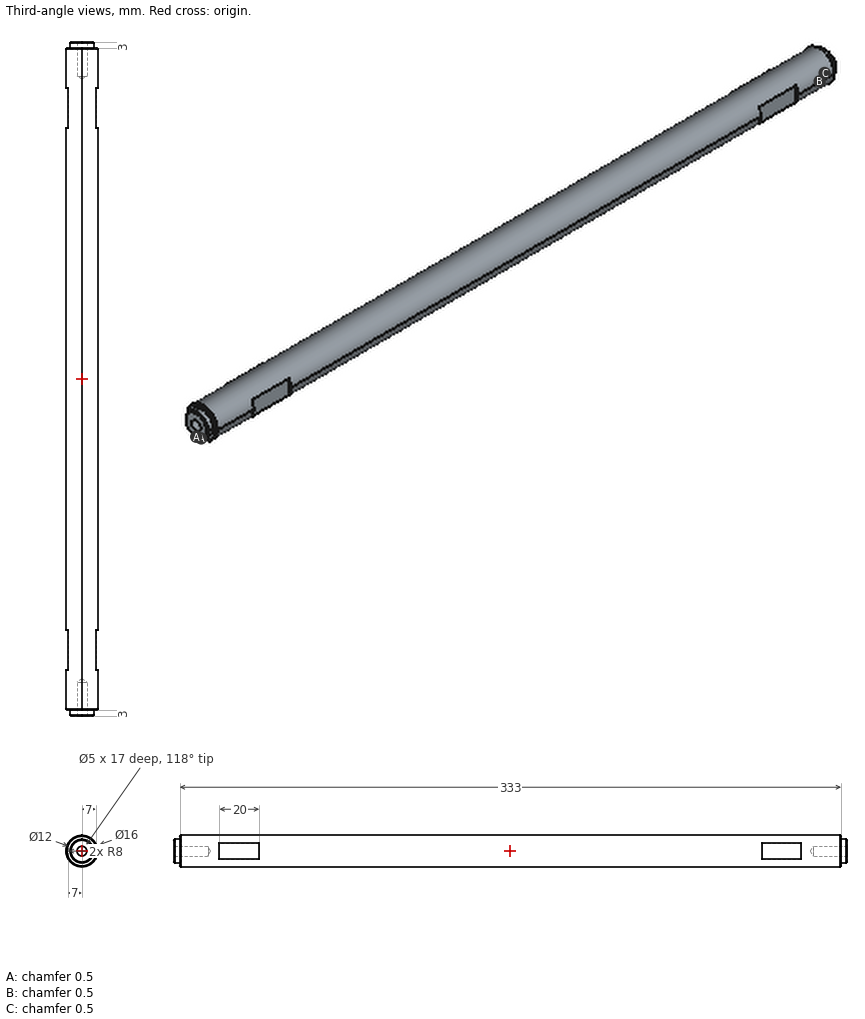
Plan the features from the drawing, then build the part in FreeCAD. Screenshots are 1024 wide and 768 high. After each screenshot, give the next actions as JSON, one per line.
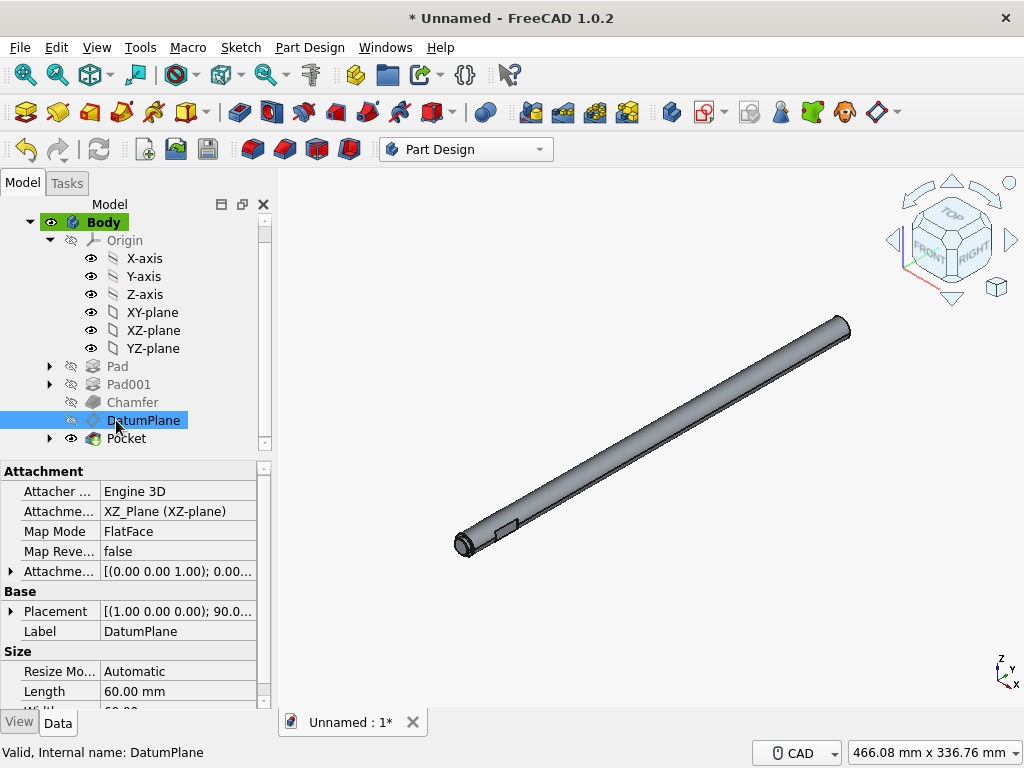
{"action": "key", "text": "2"}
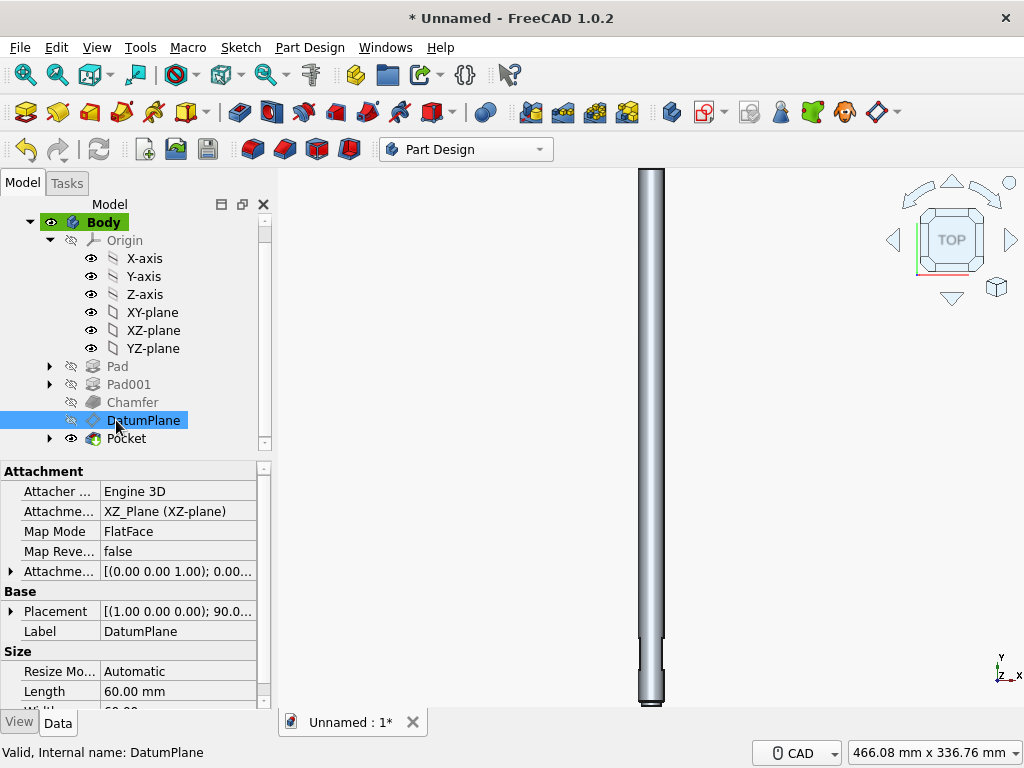
{"action": "left_click", "coordinate": [136, 330]}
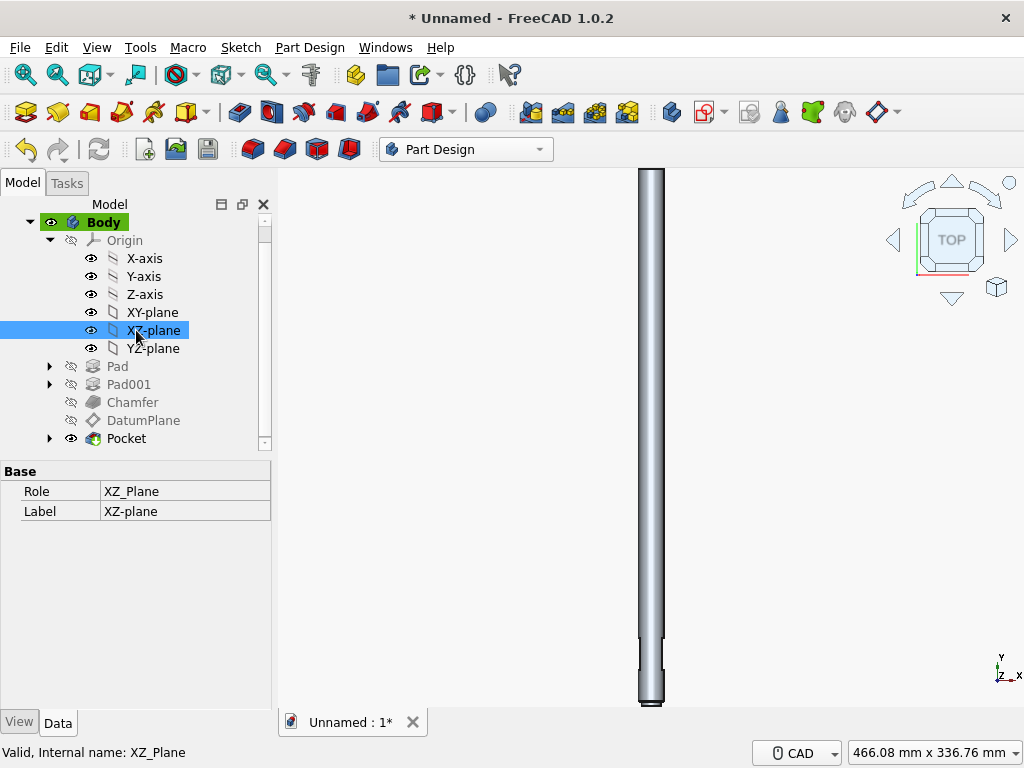
{"action": "left_click", "coordinate": [878, 112]}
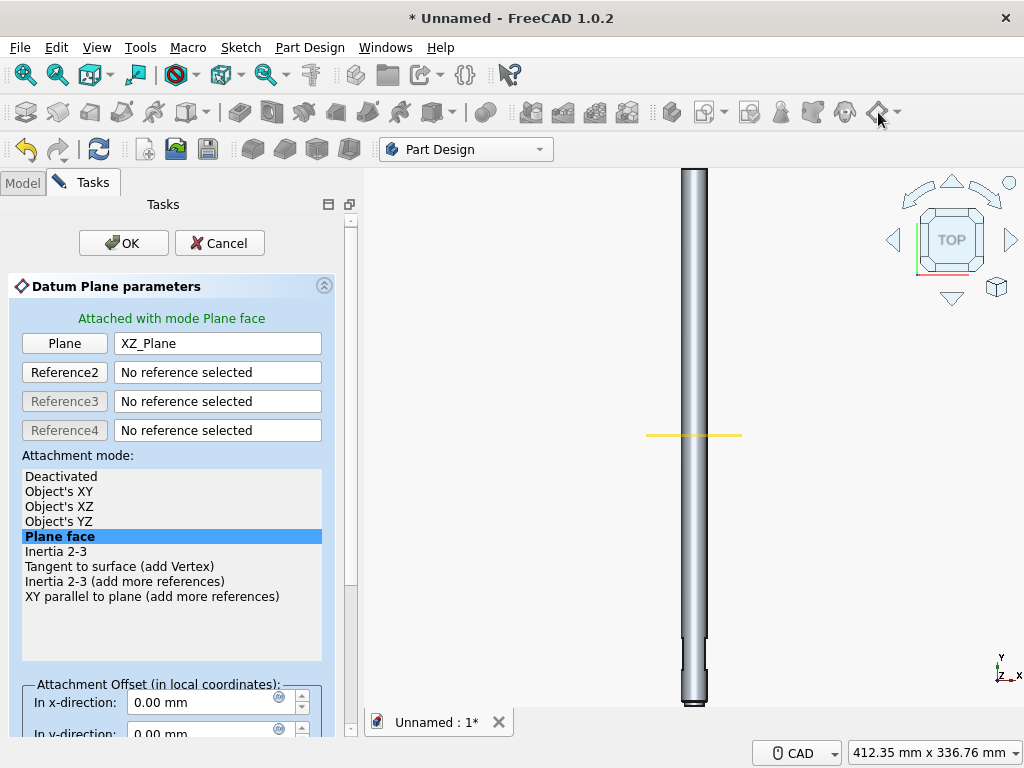
{"action": "scroll", "coordinate": [351, 475], "scroll_direction": "down", "scroll_amount": 2}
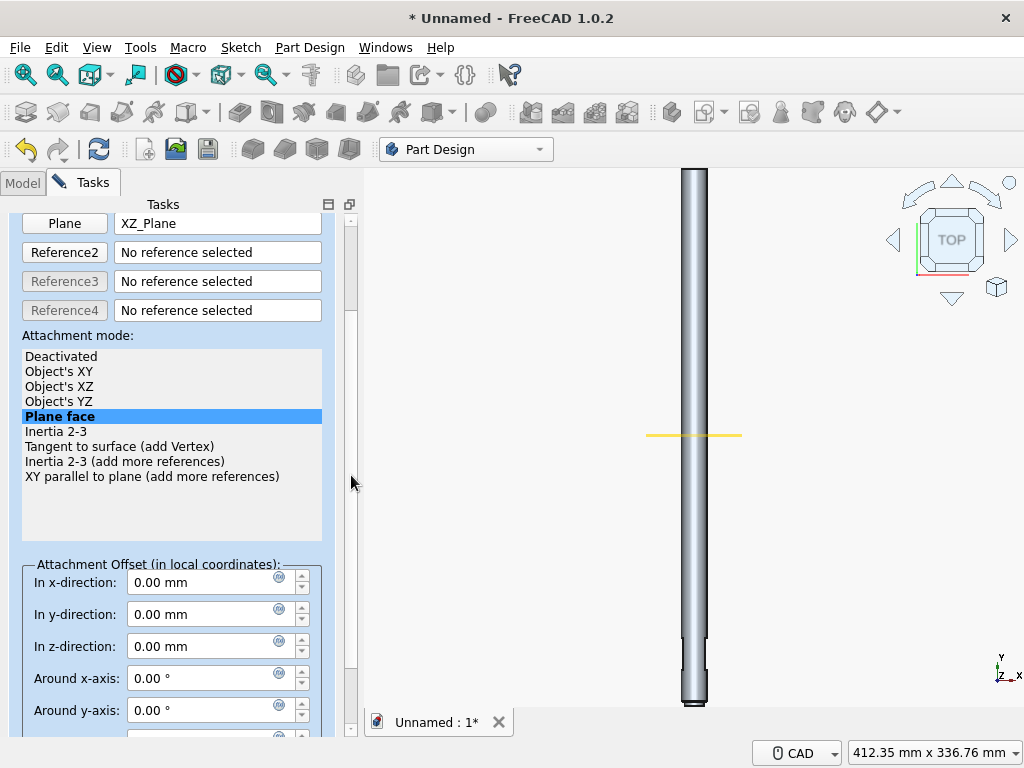
{"action": "triple_click", "coordinate": [210, 646]}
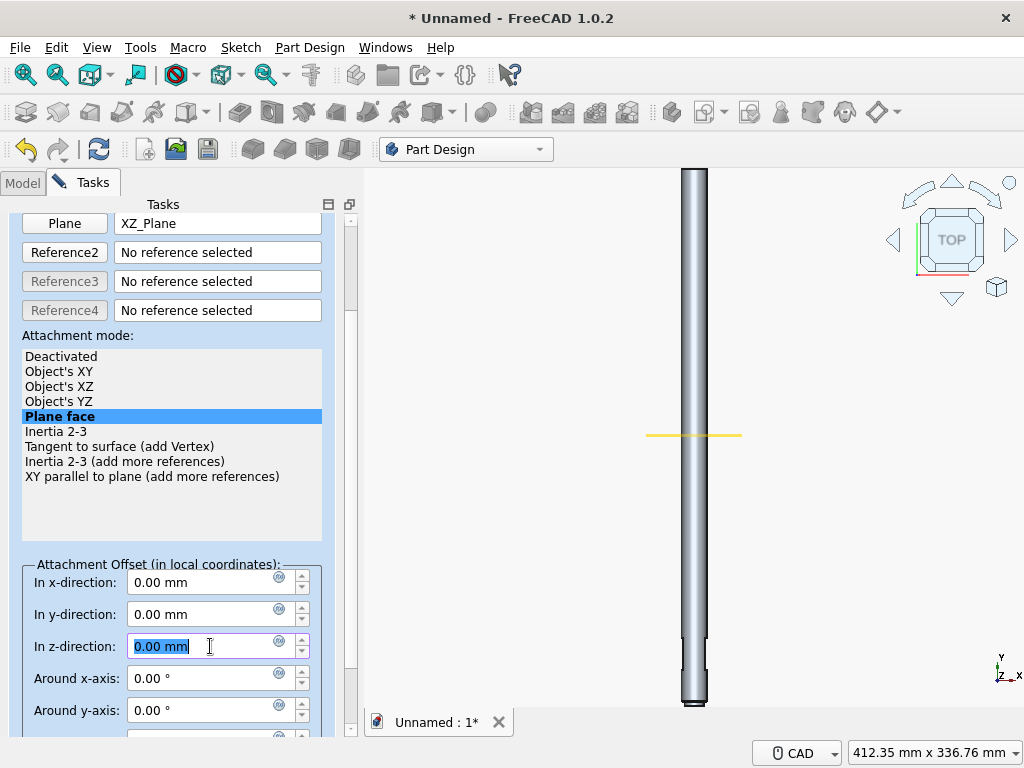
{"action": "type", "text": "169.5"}
{"action": "key", "text": "Tab"}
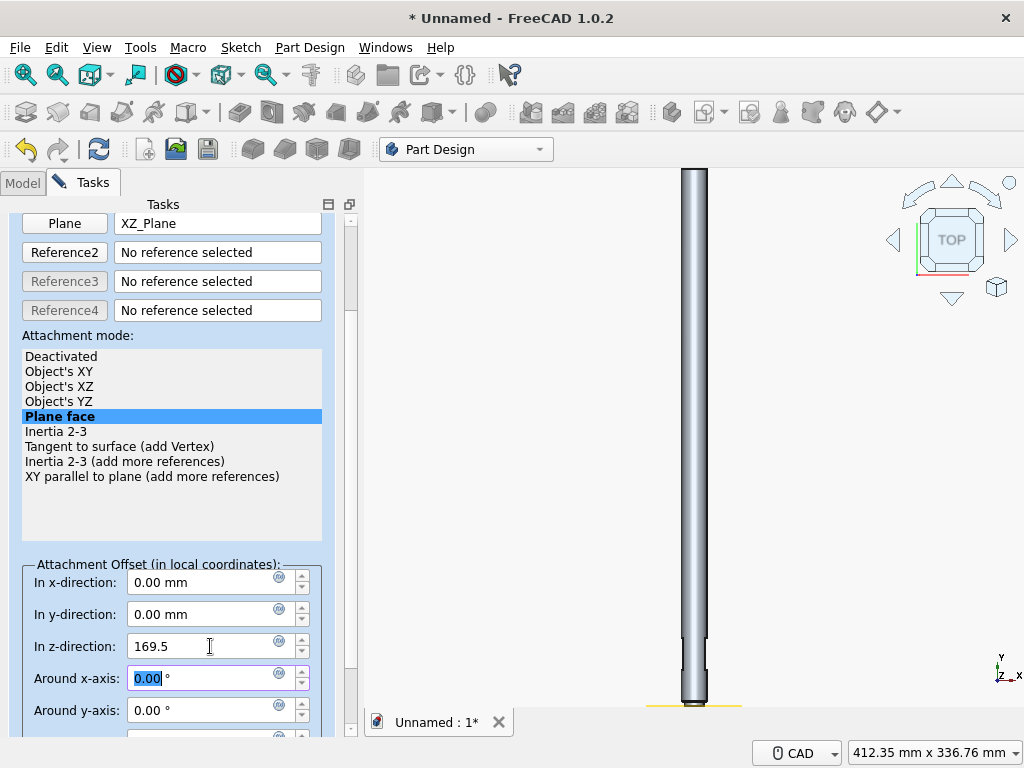
{"action": "scroll", "coordinate": [351, 475], "scroll_direction": "up", "scroll_amount": 3}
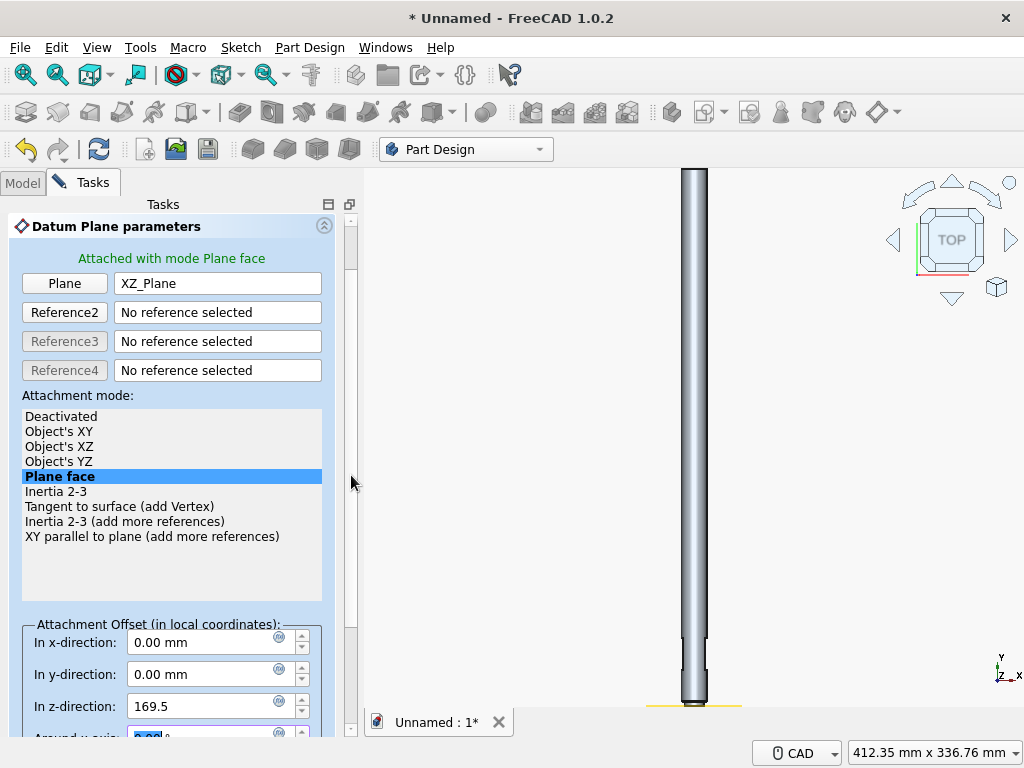
{"action": "left_click", "coordinate": [124, 243]}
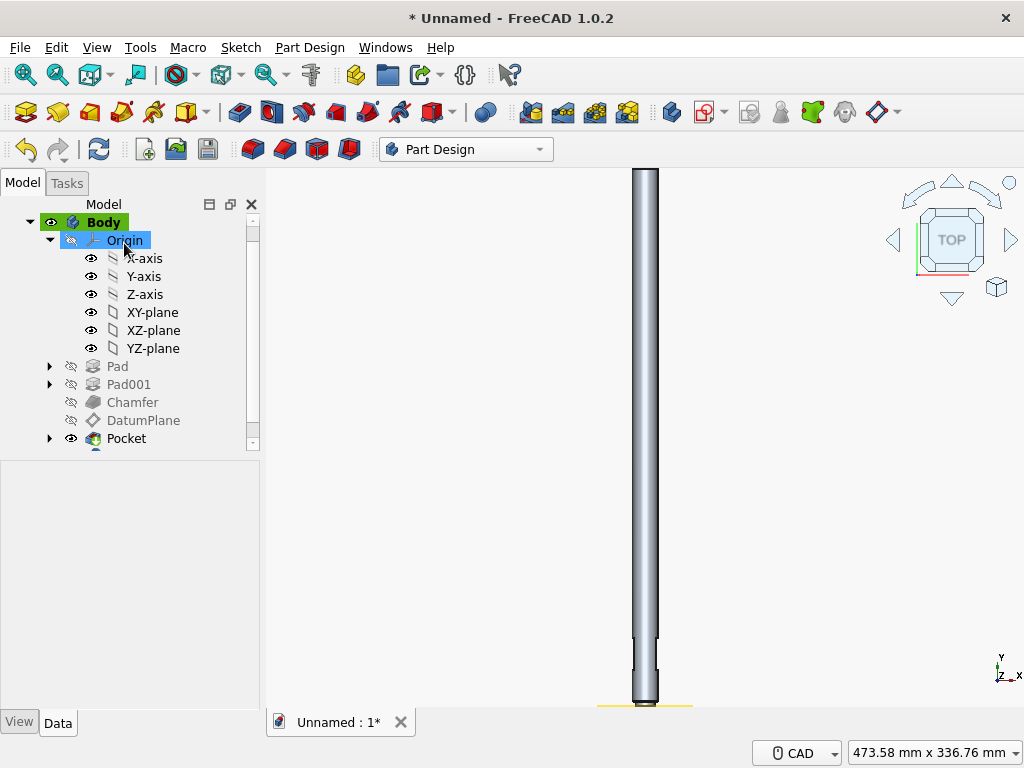
{"action": "scroll", "coordinate": [120, 326], "scroll_direction": "down", "scroll_amount": 3}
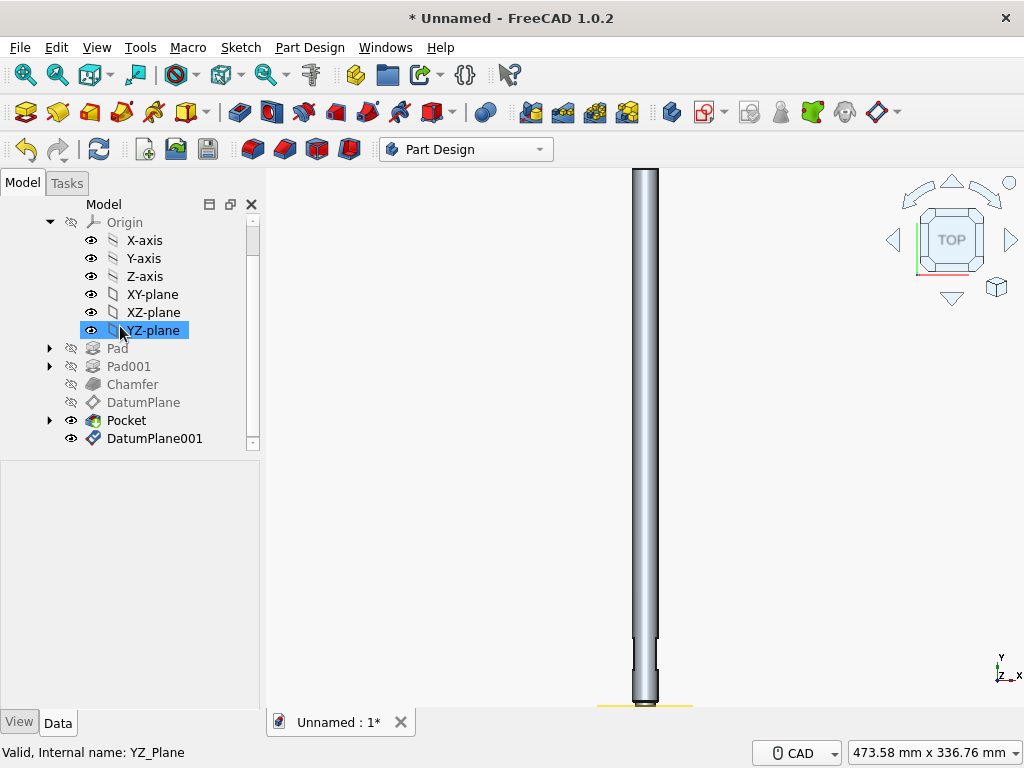
{"action": "left_click", "coordinate": [116, 438]}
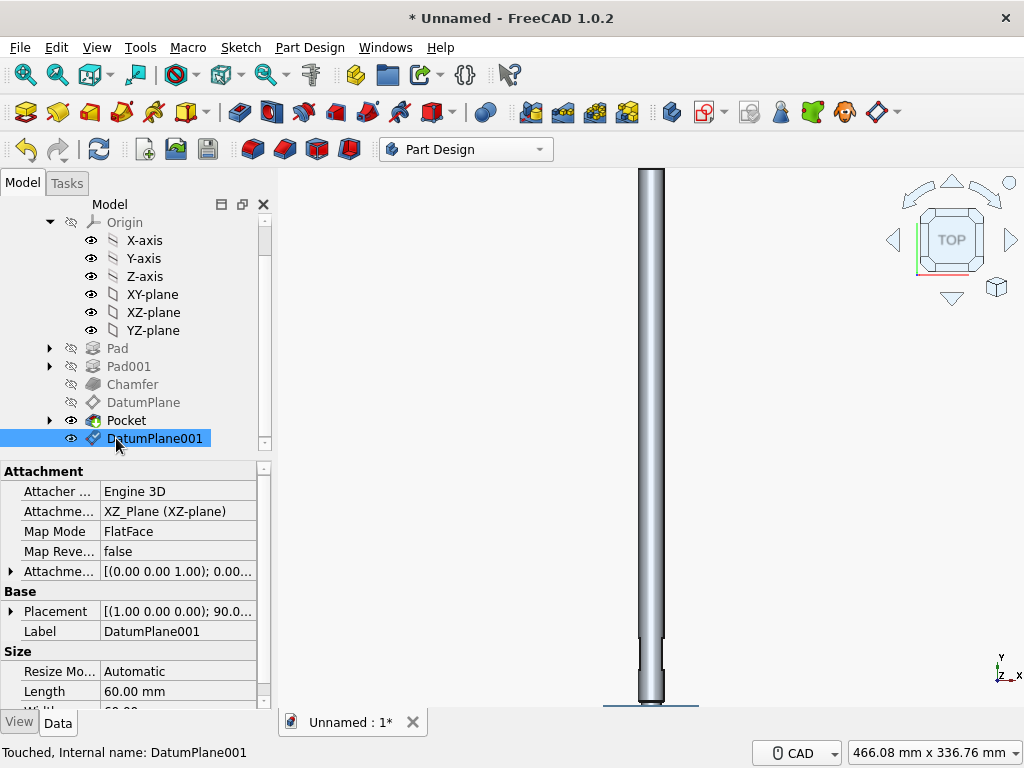
{"action": "left_click", "coordinate": [704, 112]}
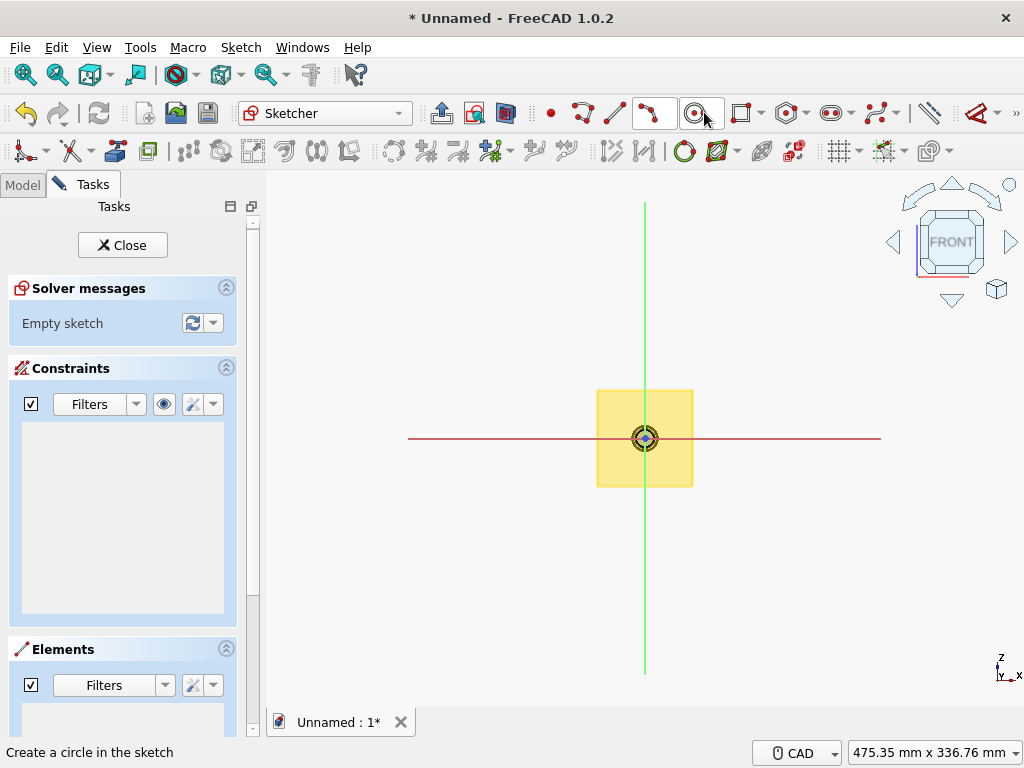
{"action": "scroll", "coordinate": [649, 438], "scroll_direction": "up", "scroll_amount": 15}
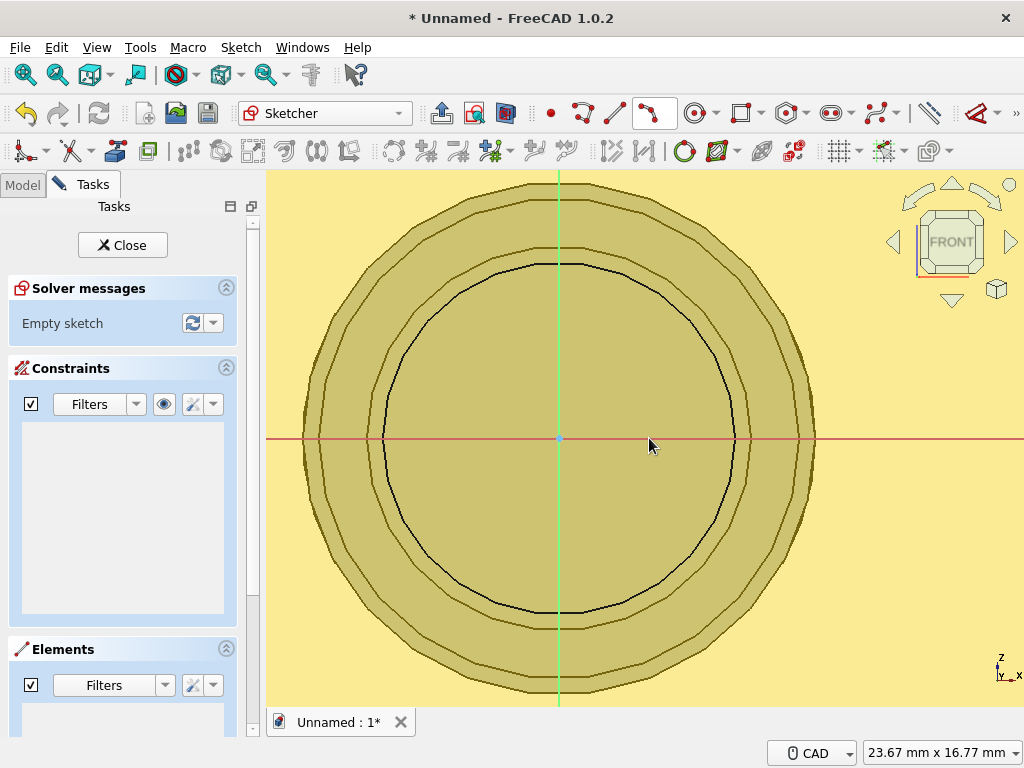
{"action": "scroll", "coordinate": [545, 438], "scroll_direction": "up", "scroll_amount": 4}